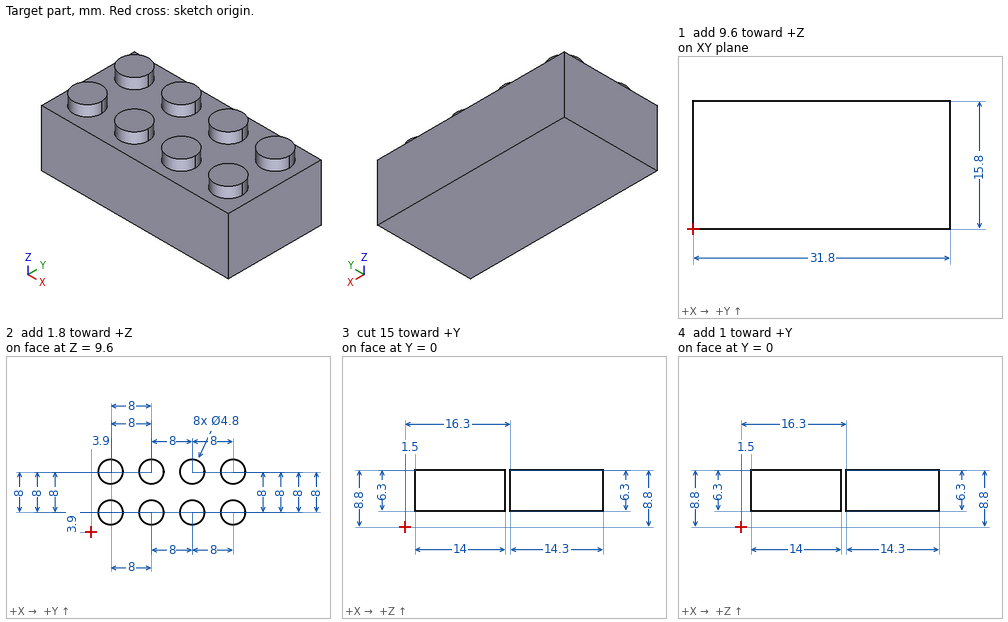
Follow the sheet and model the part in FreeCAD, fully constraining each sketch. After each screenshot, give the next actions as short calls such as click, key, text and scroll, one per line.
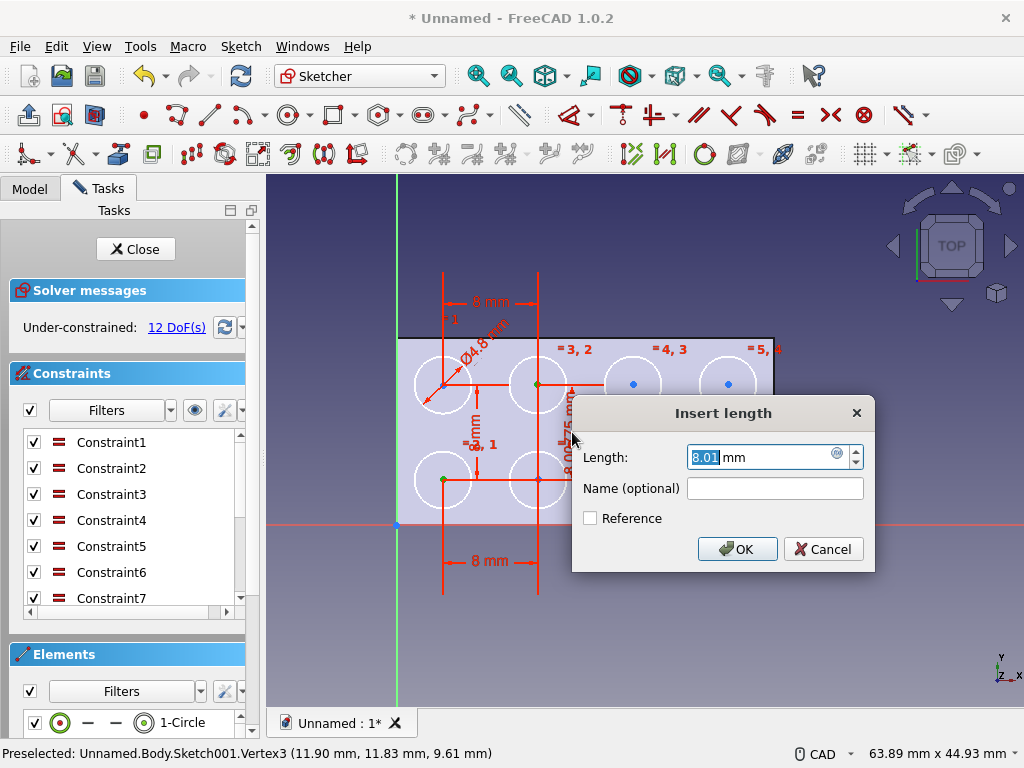
text(8)
key(Return)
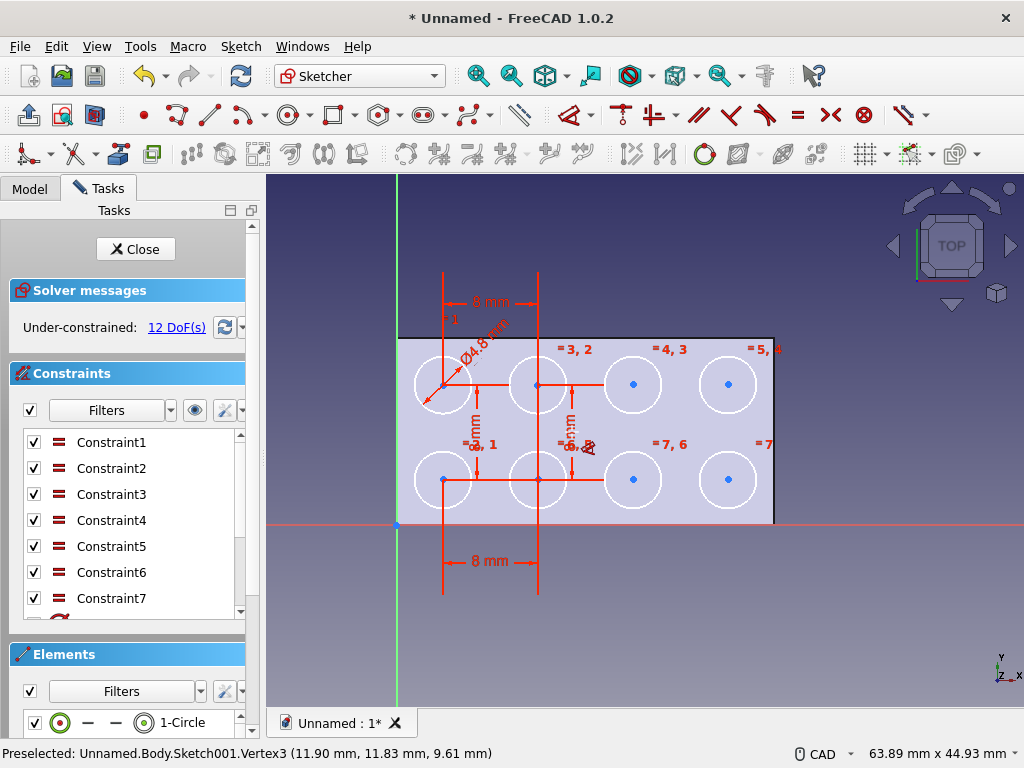
click(538, 385)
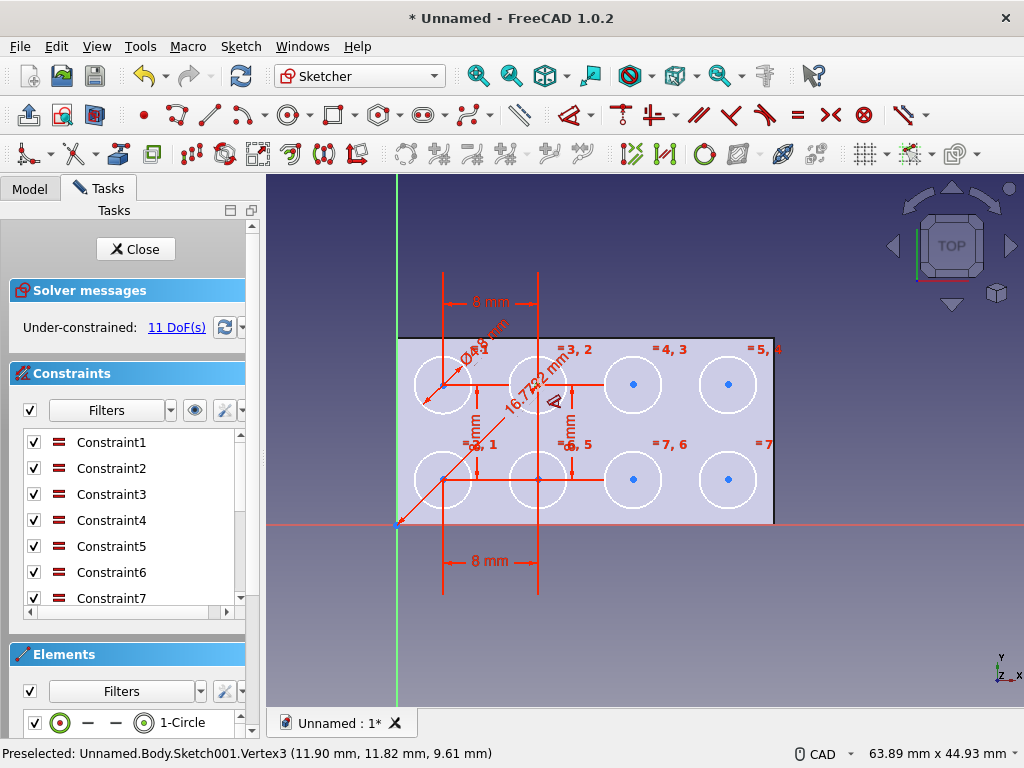
click(633, 385)
click(585, 351)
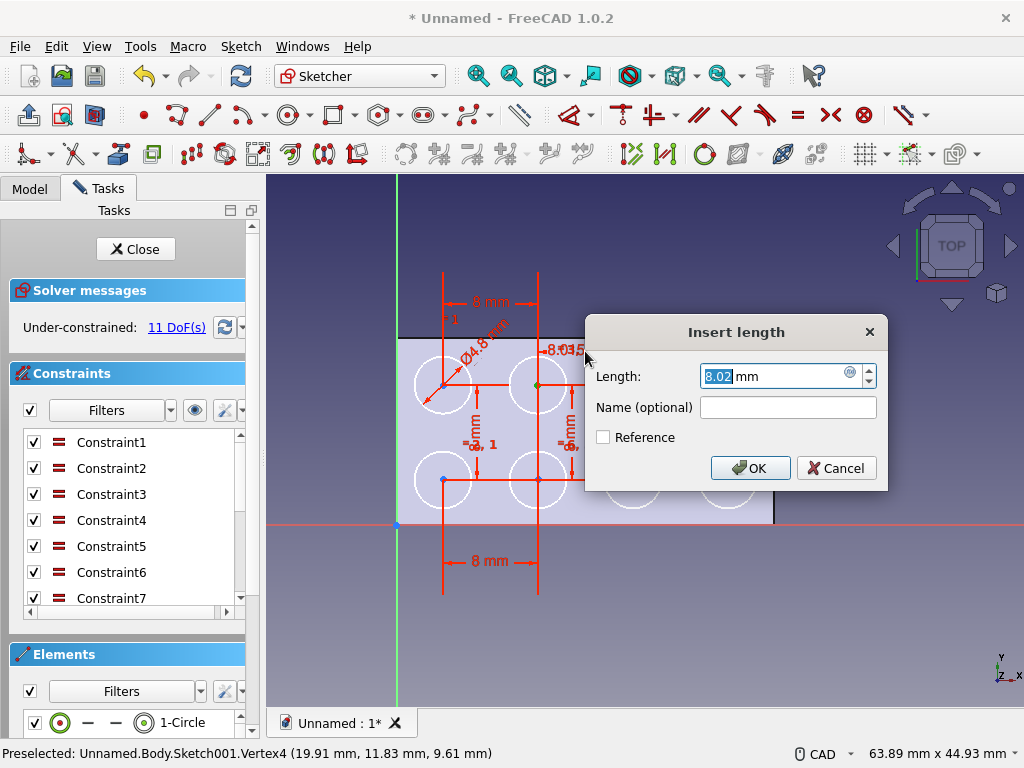
text(8)
key(Return)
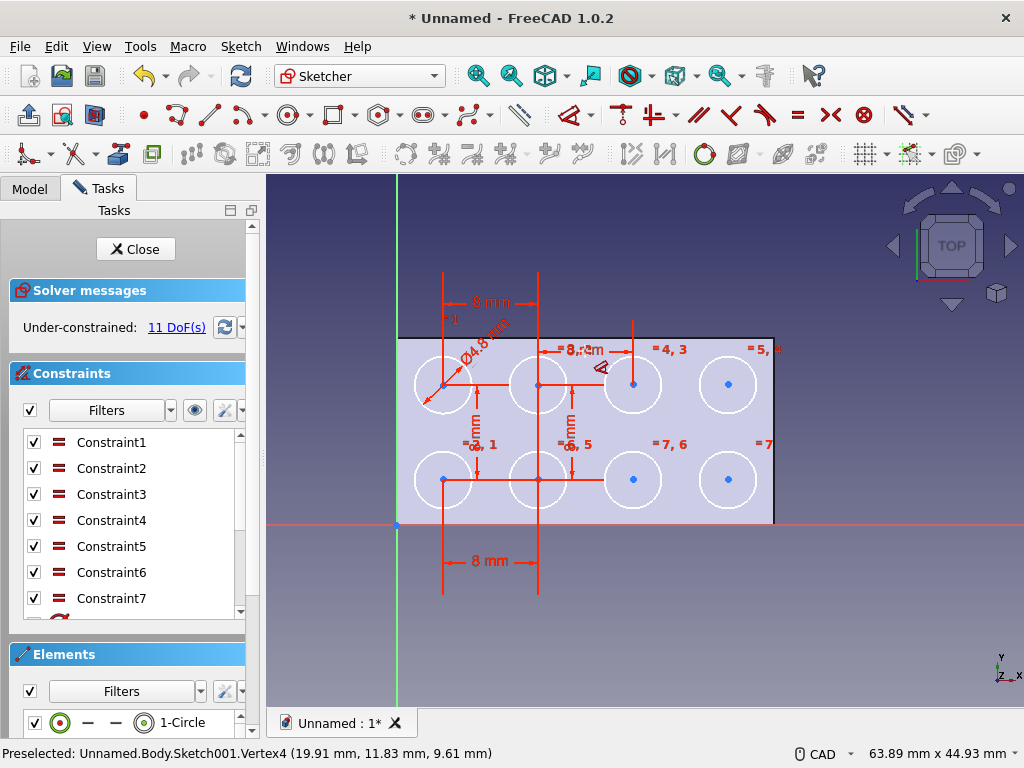
click(443, 480)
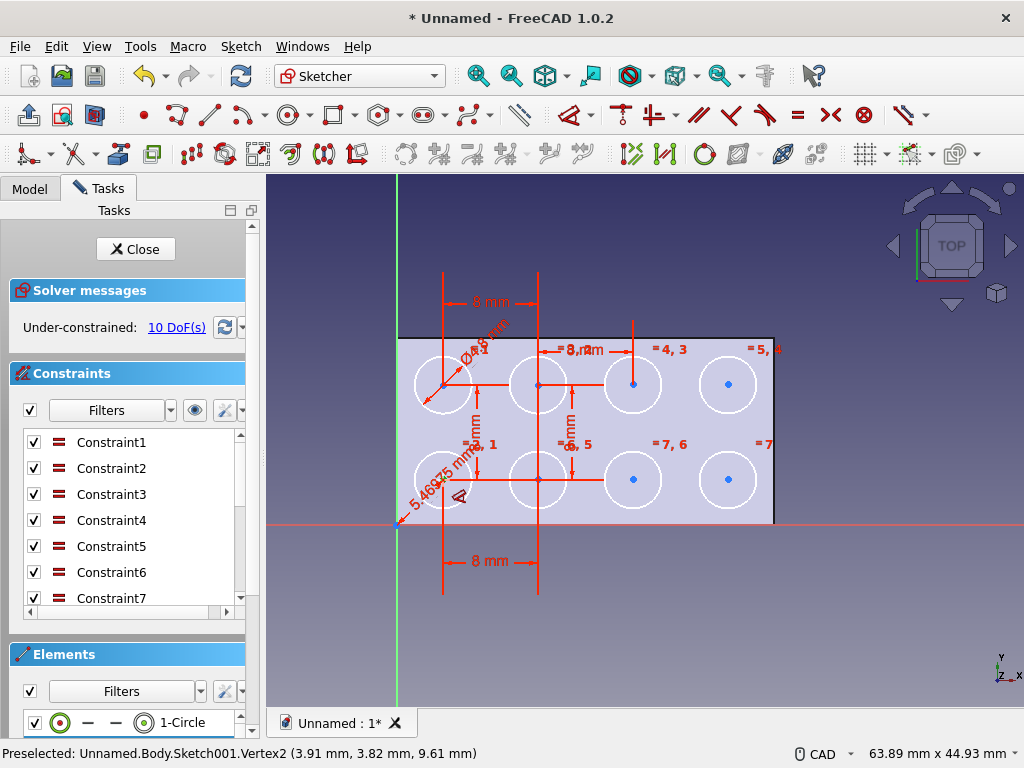
click(633, 385)
click(667, 432)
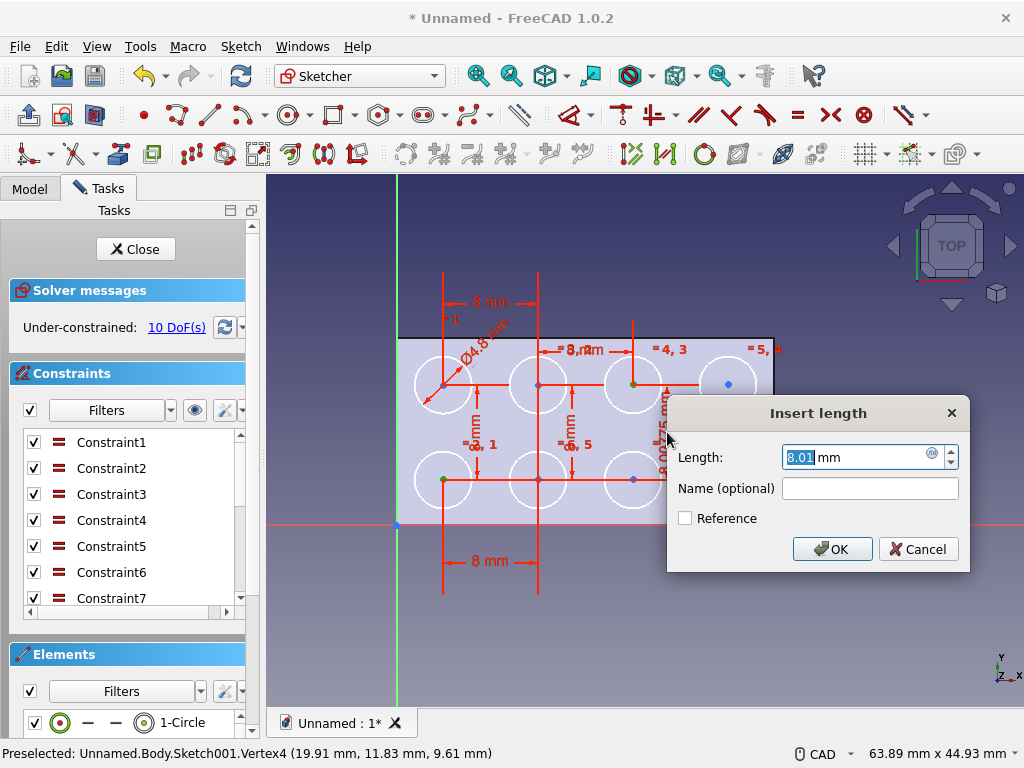
text(8)
key(Return)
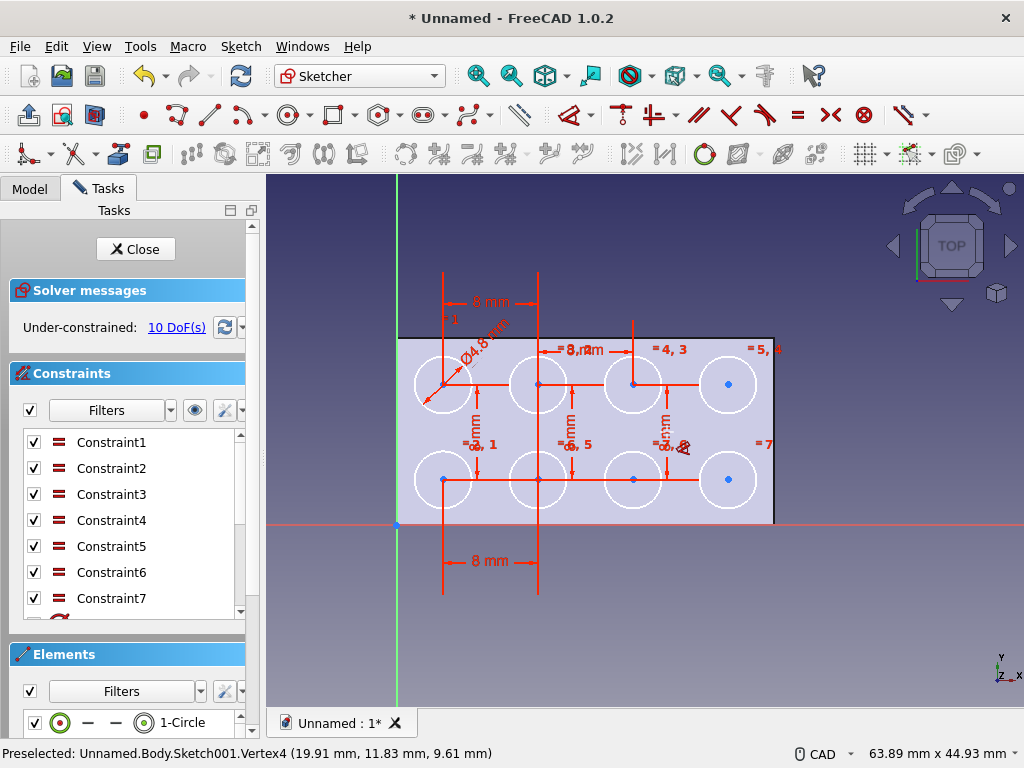
click(633, 385)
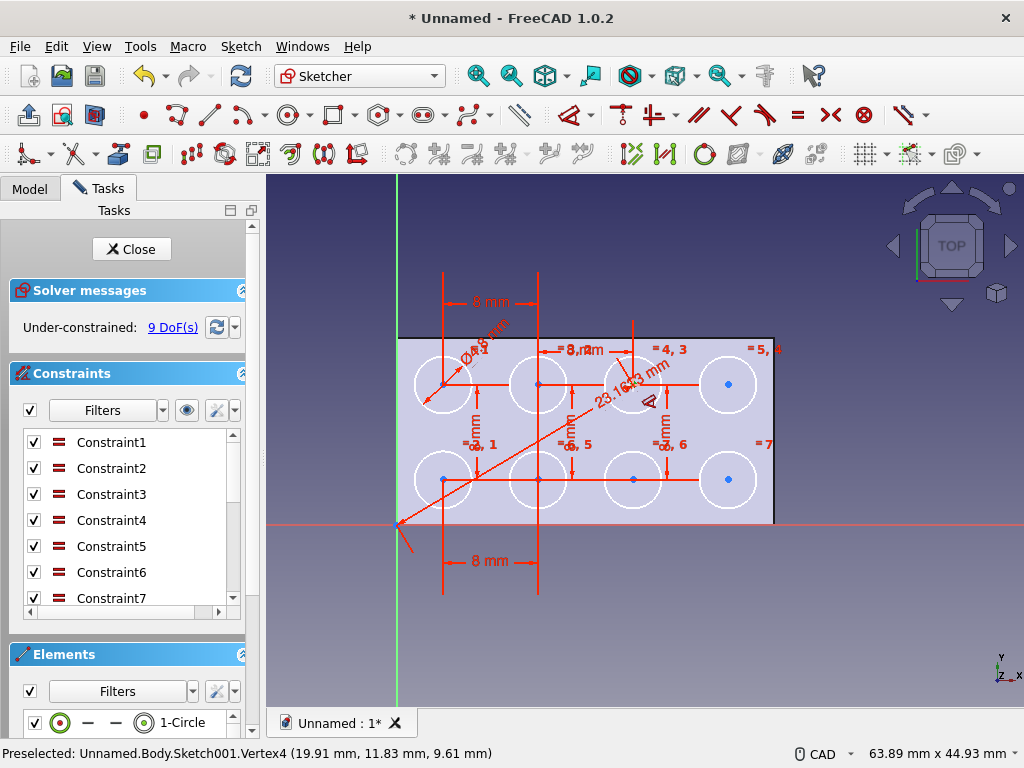
click(728, 385)
click(681, 351)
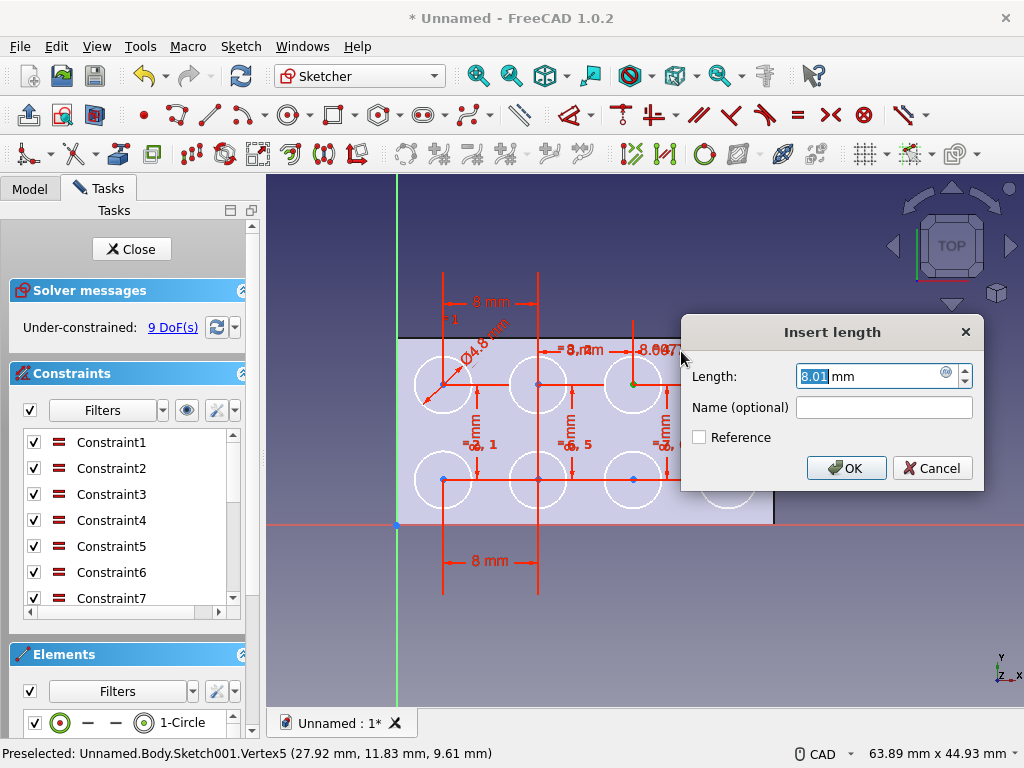
text(8)
key(Return)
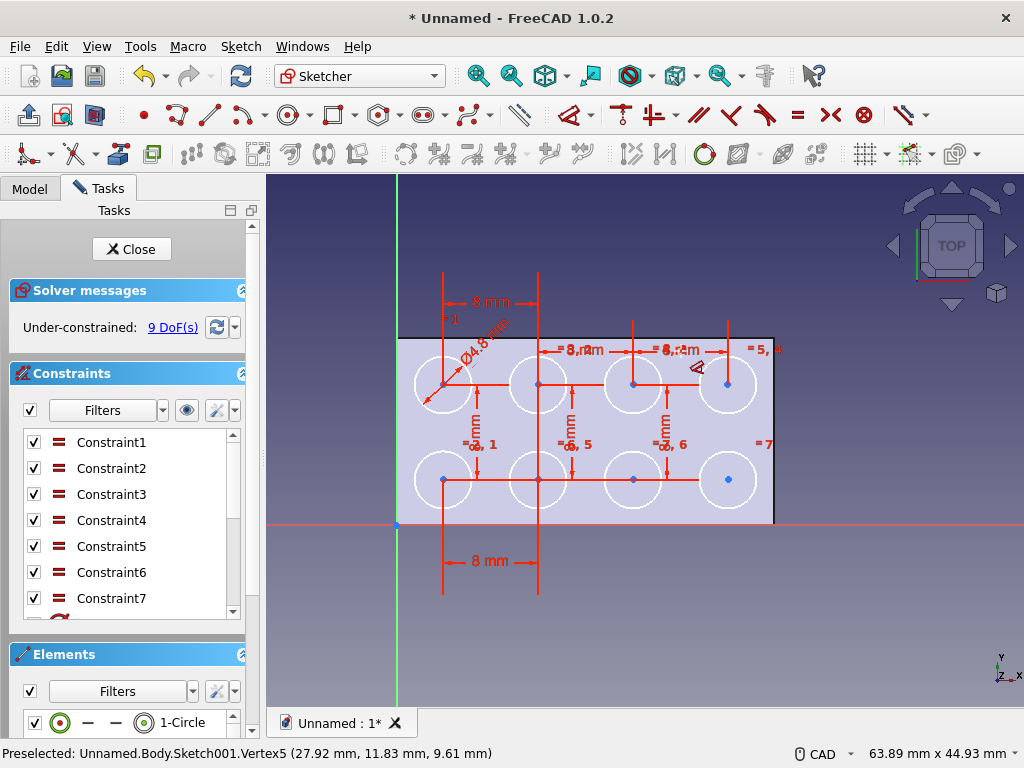
click(443, 480)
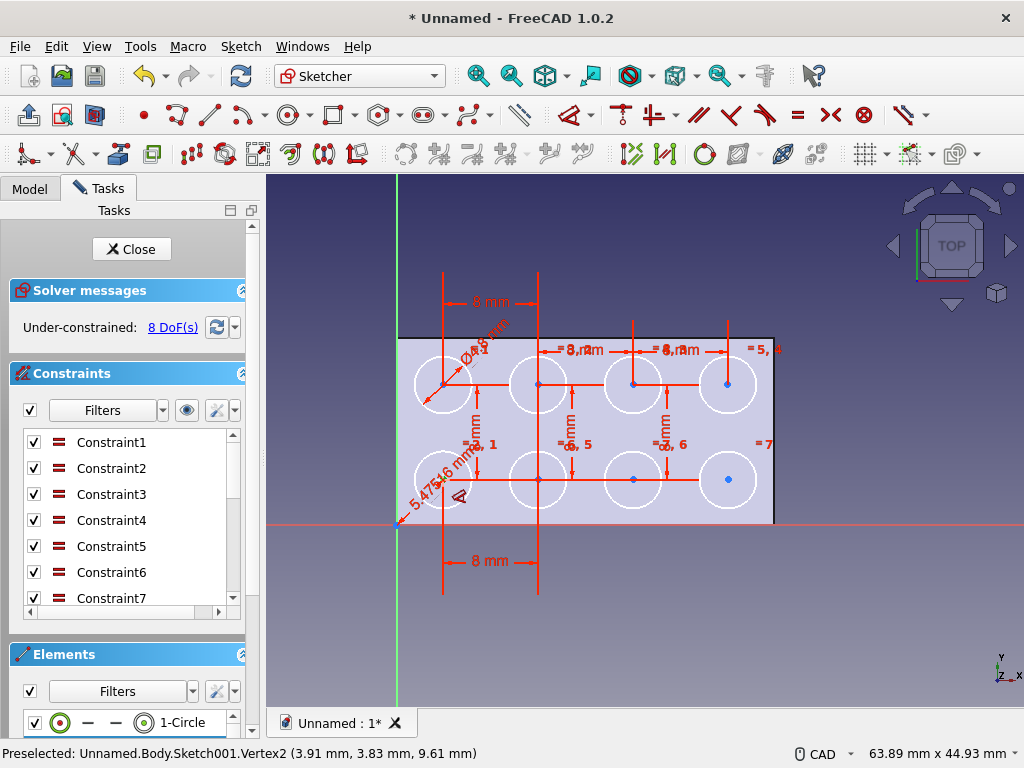
click(728, 385)
click(762, 432)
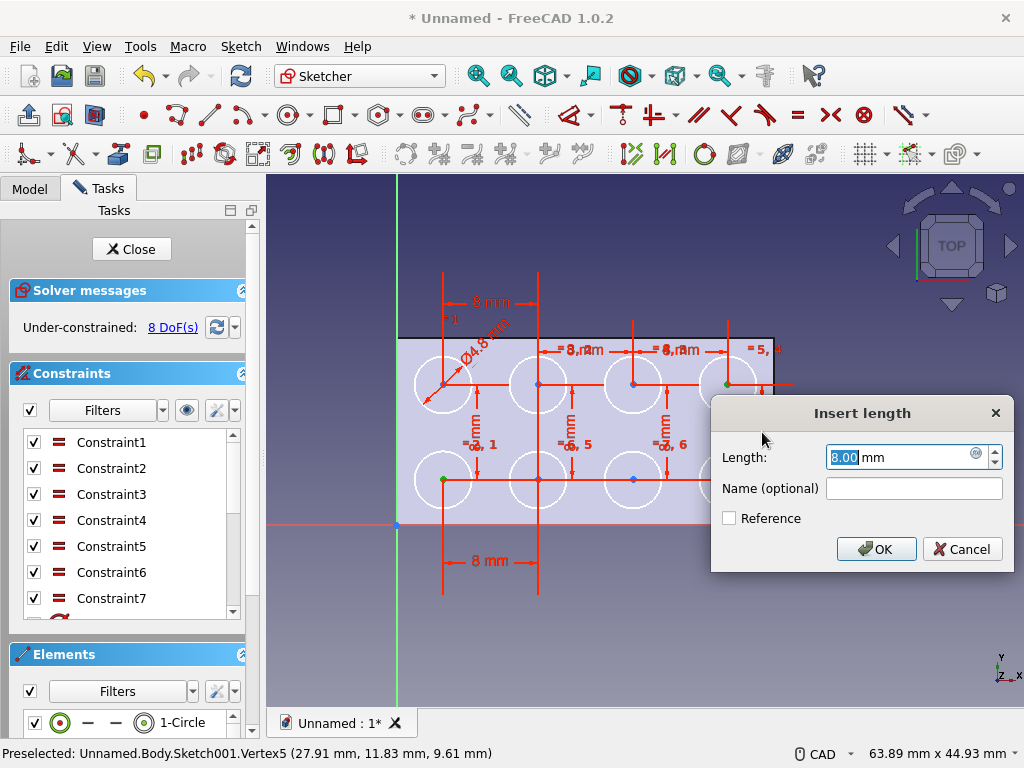
text(8)
key(Return)